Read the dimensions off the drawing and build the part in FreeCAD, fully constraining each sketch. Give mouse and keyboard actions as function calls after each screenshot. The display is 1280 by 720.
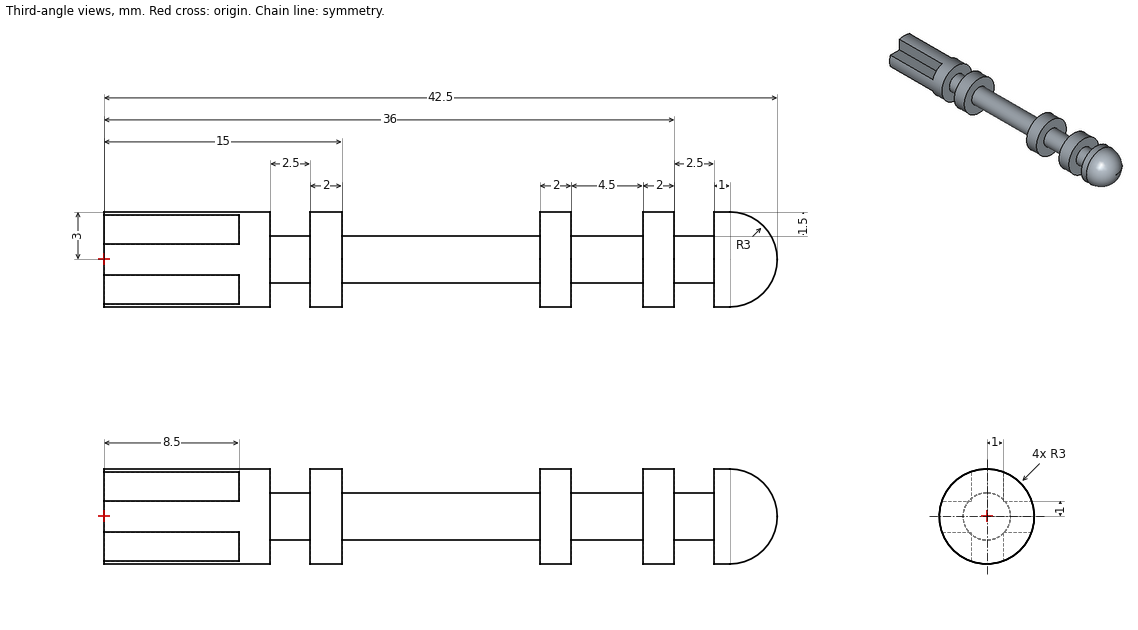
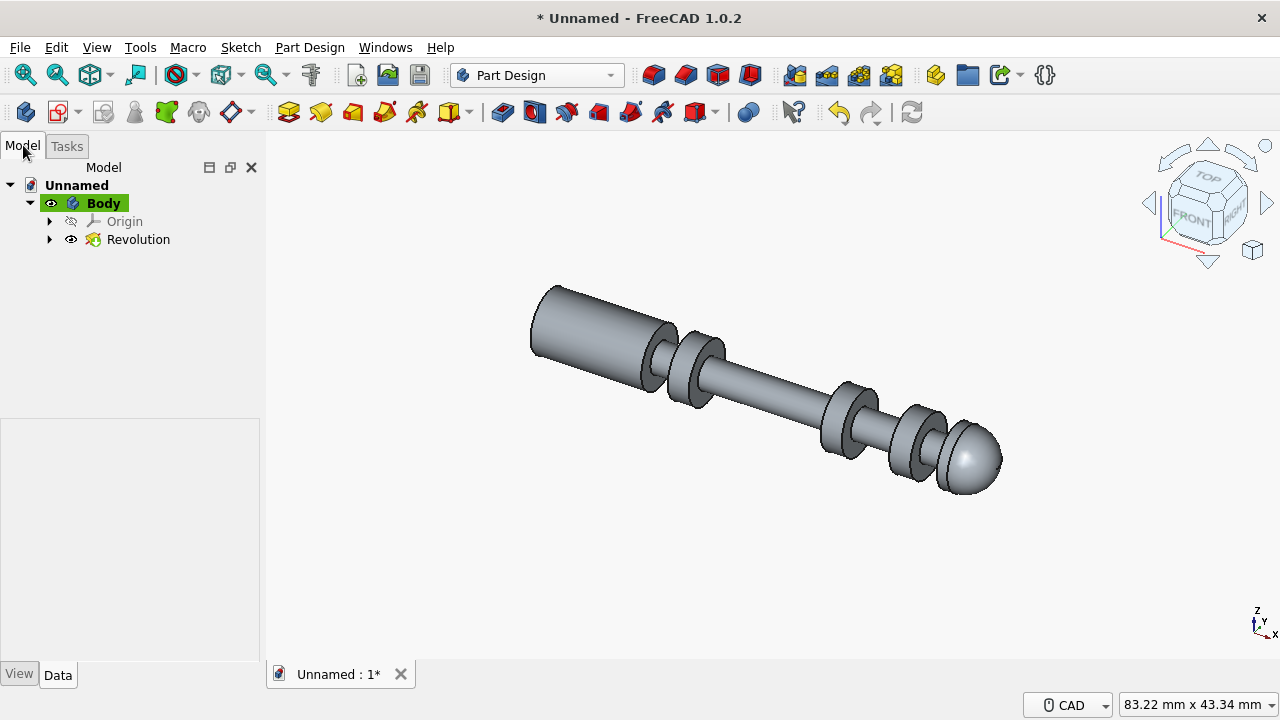
click(50, 221)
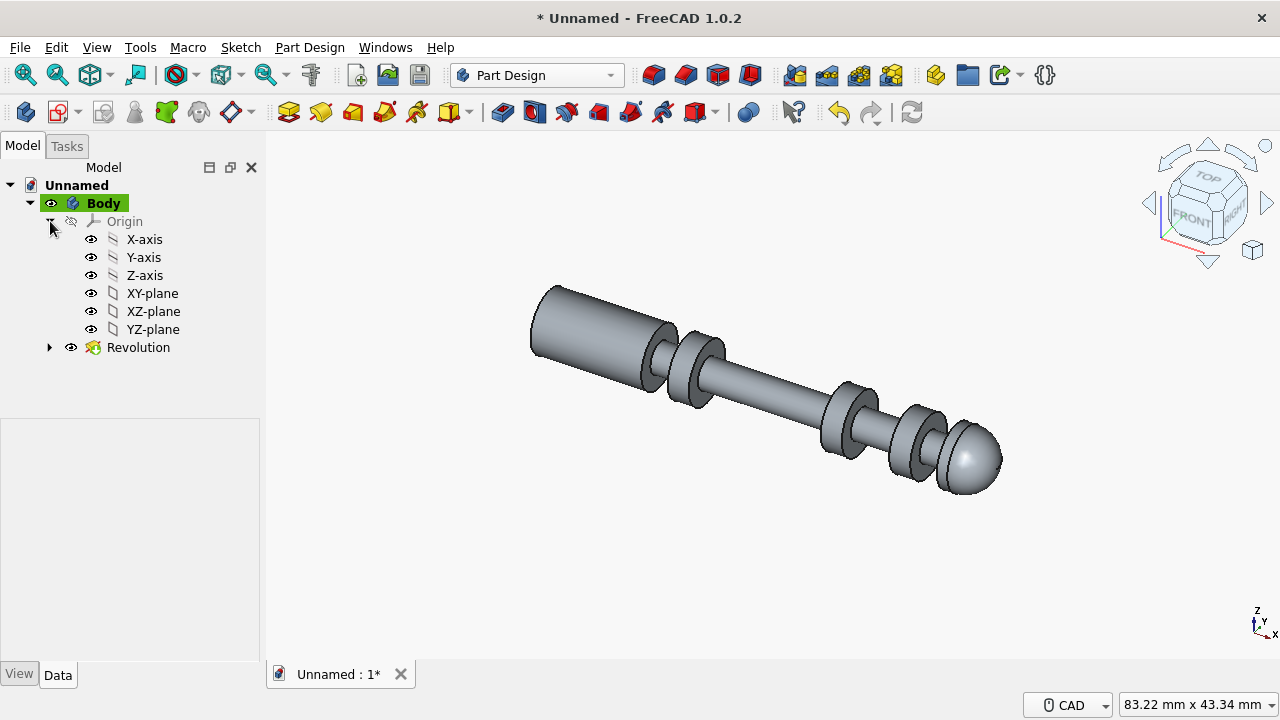
click(136, 329)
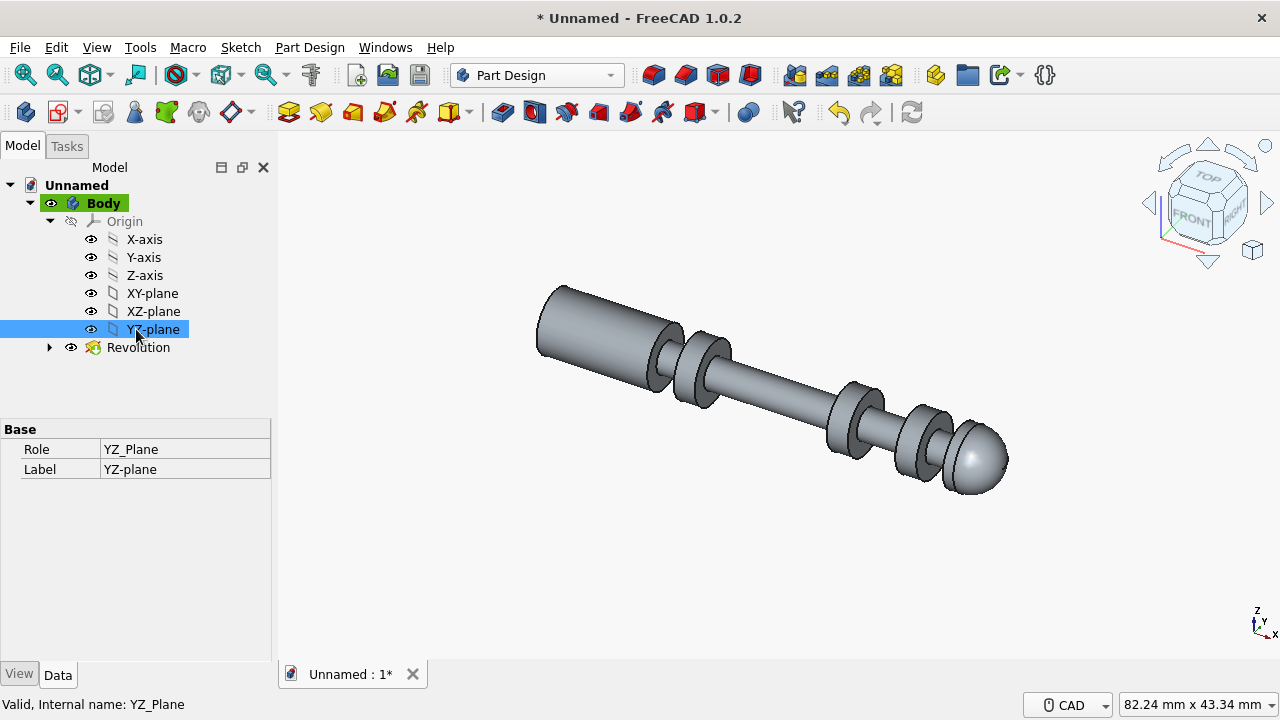
click(232, 112)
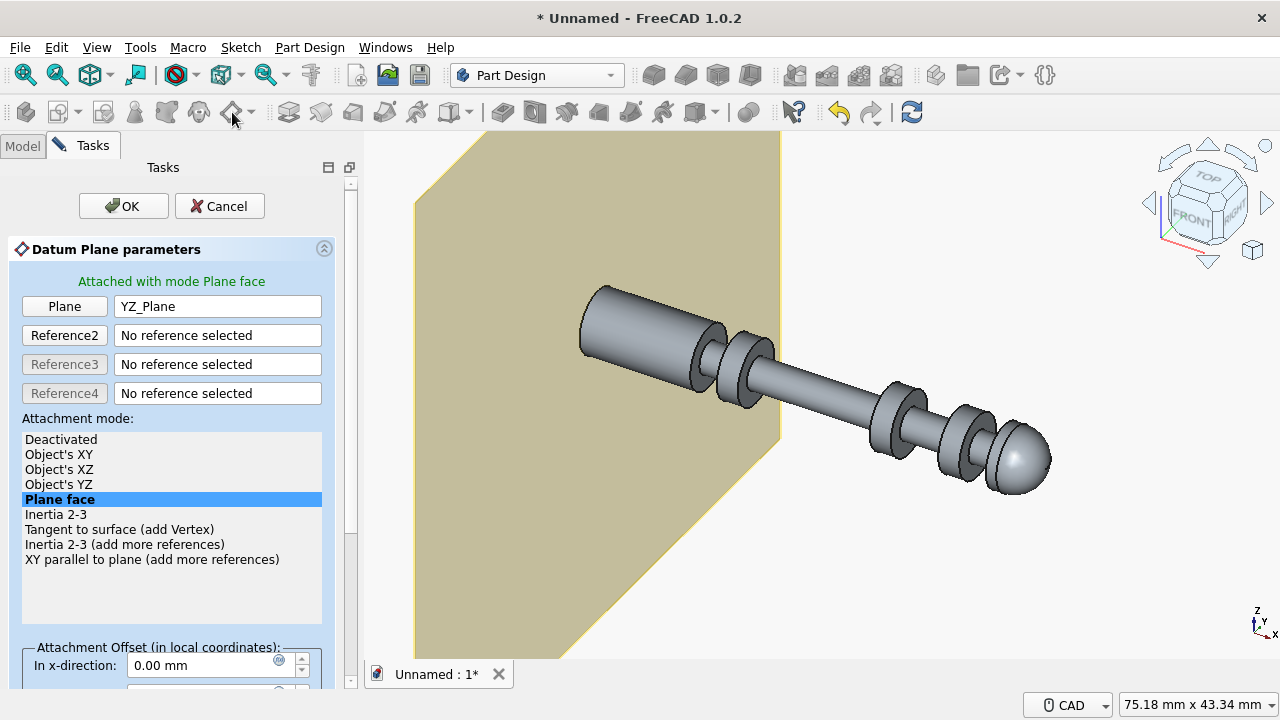
scroll(351, 432, down, 2)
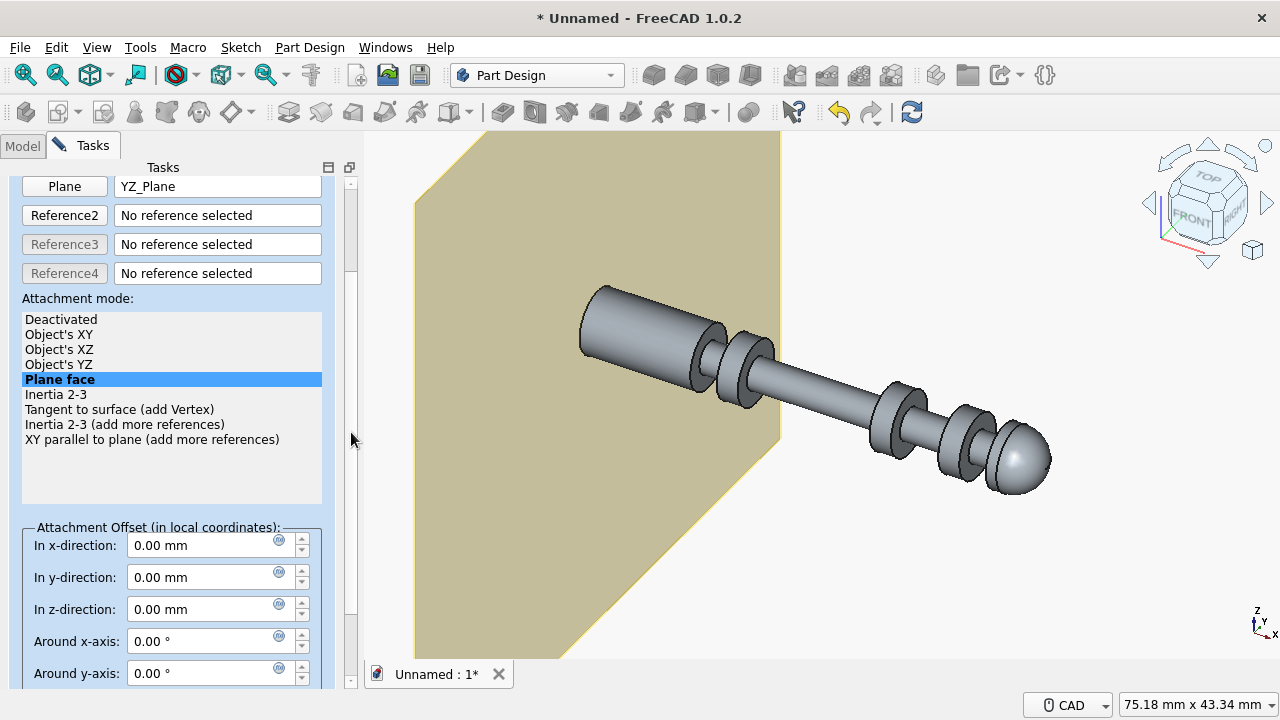
triple_click(210, 609)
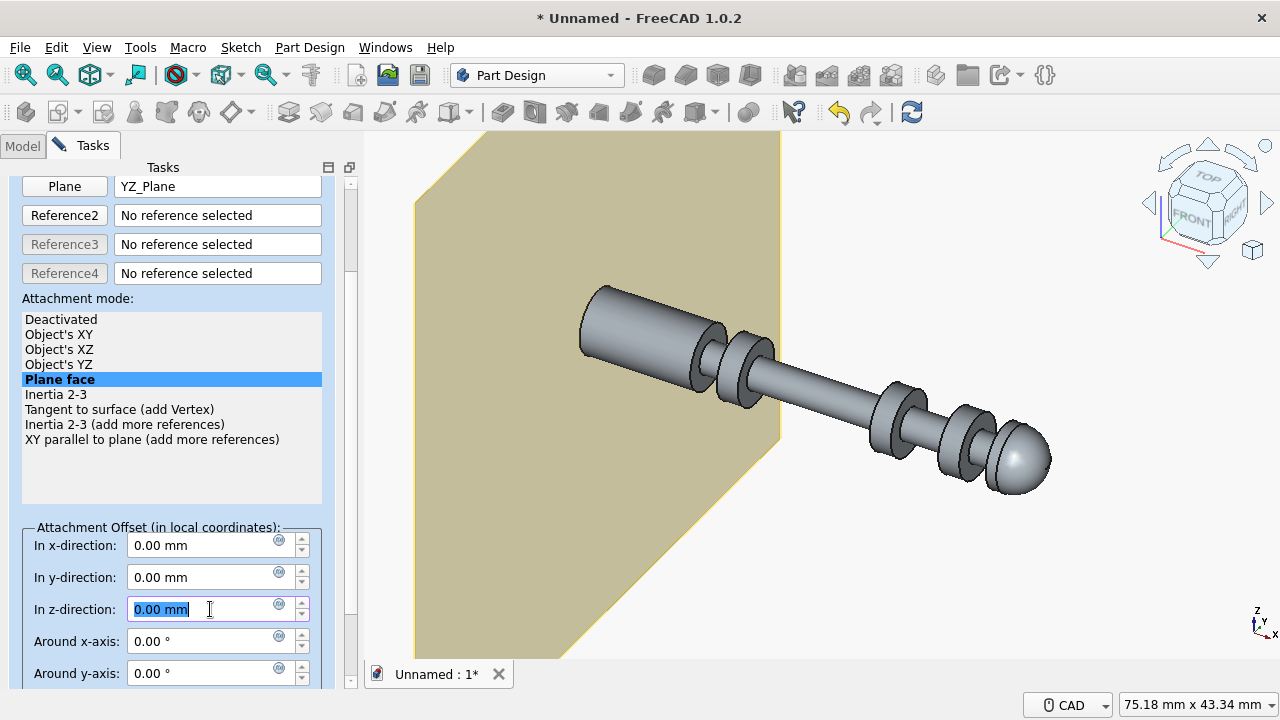
text(8.5)
key(Tab)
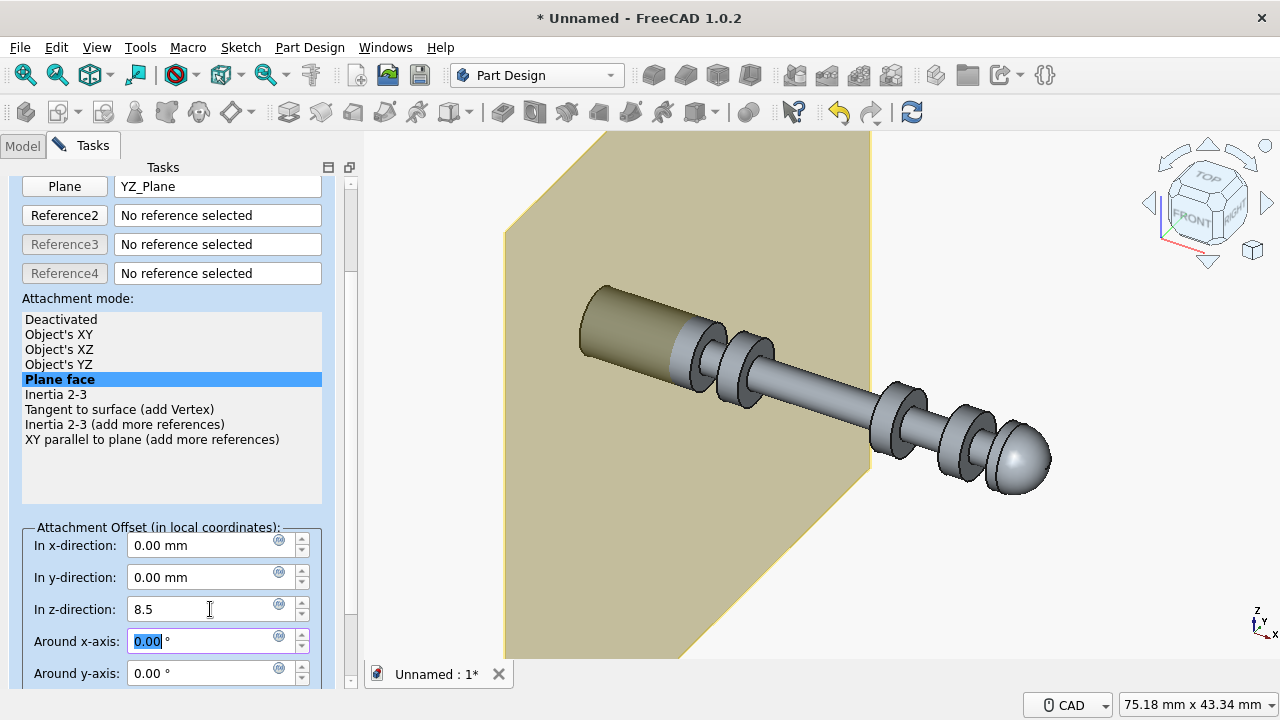
scroll(351, 432, up, 3)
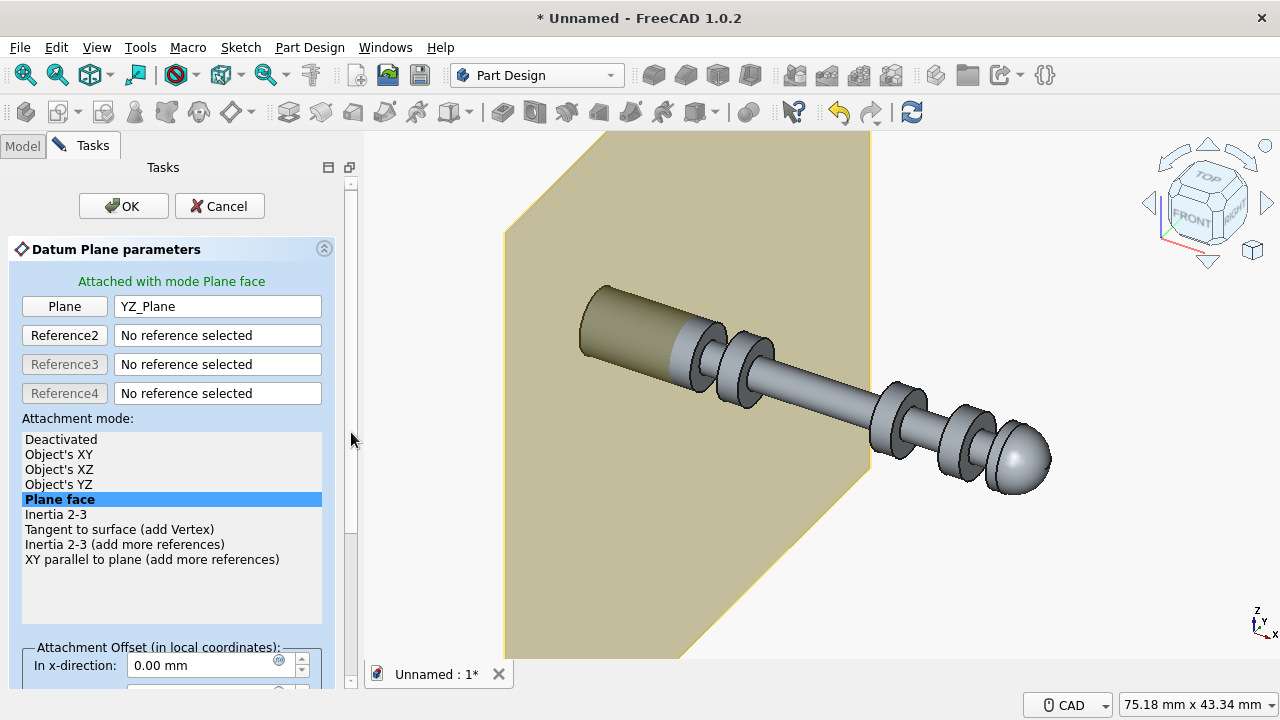
click(124, 206)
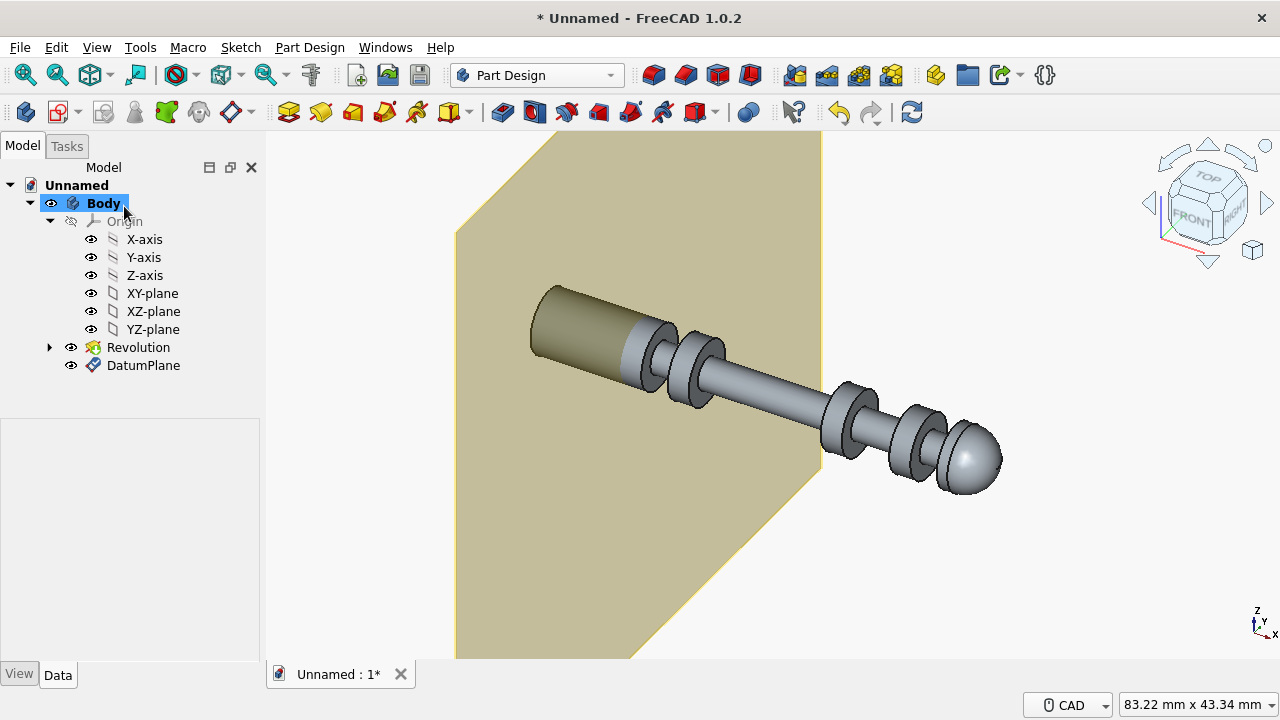
click(116, 365)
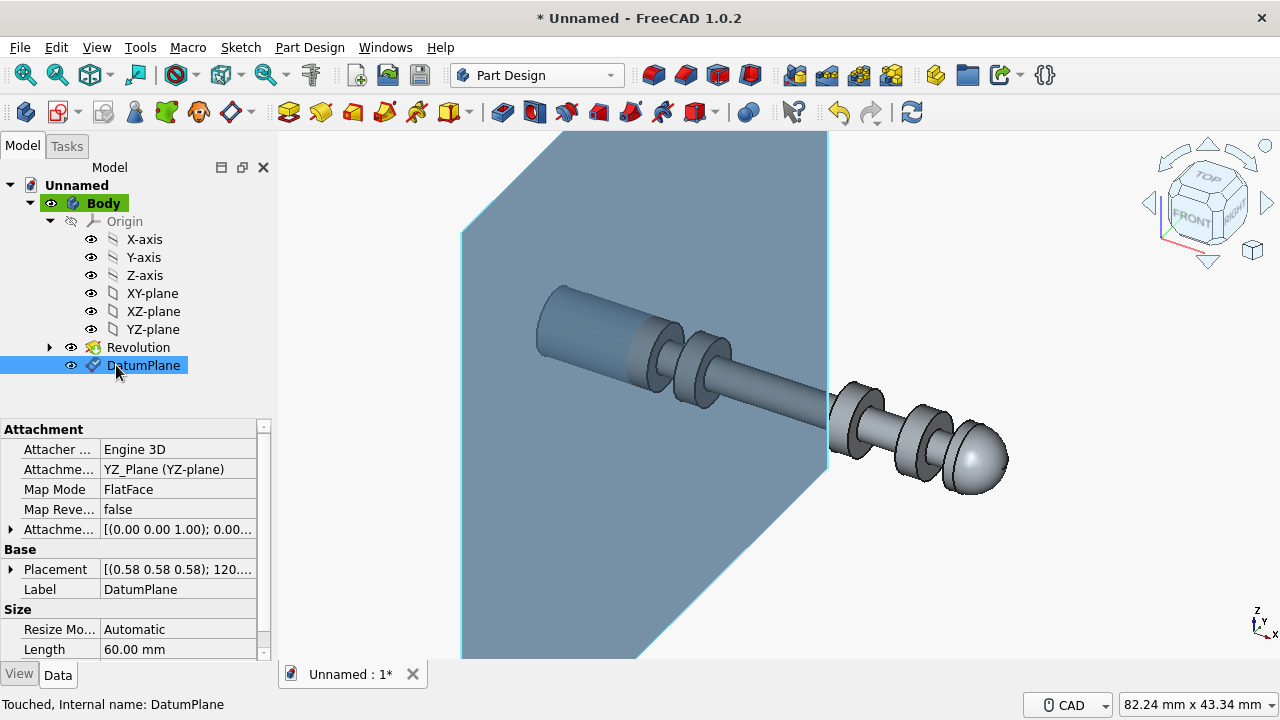
click(58, 112)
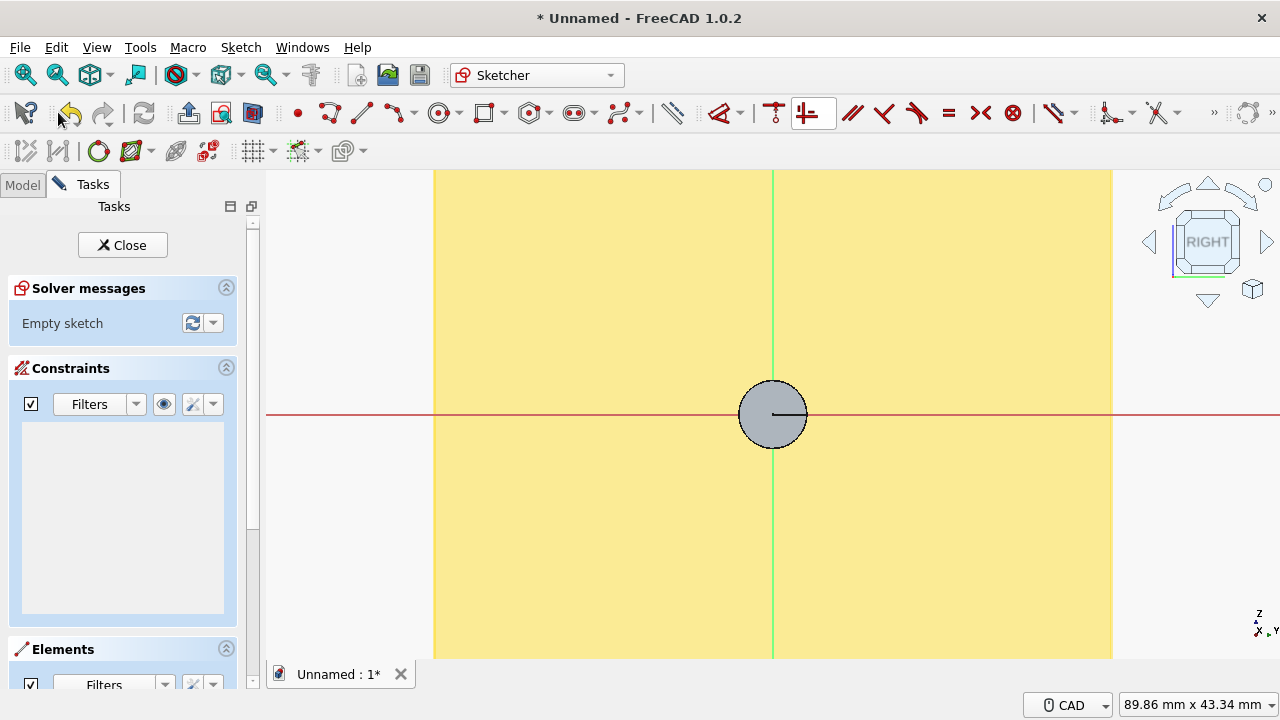
click(254, 114)